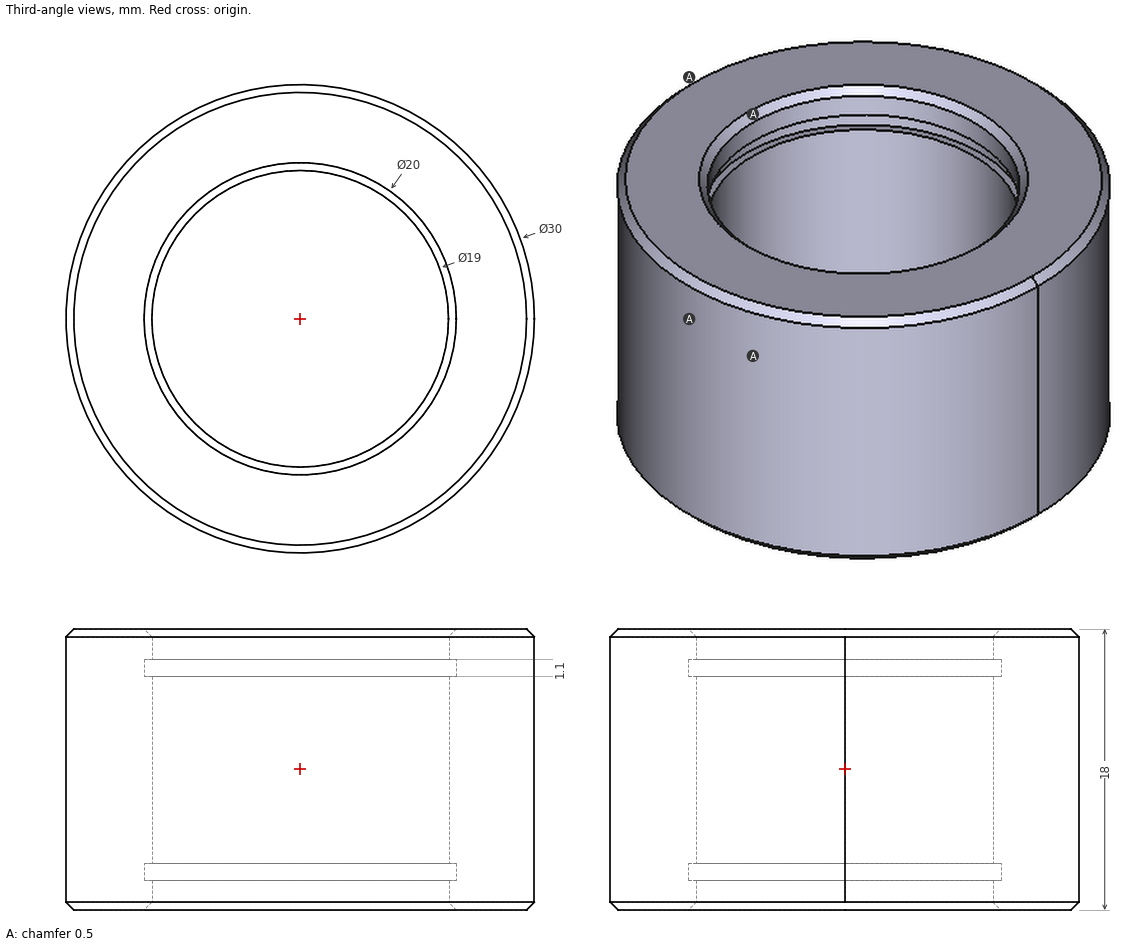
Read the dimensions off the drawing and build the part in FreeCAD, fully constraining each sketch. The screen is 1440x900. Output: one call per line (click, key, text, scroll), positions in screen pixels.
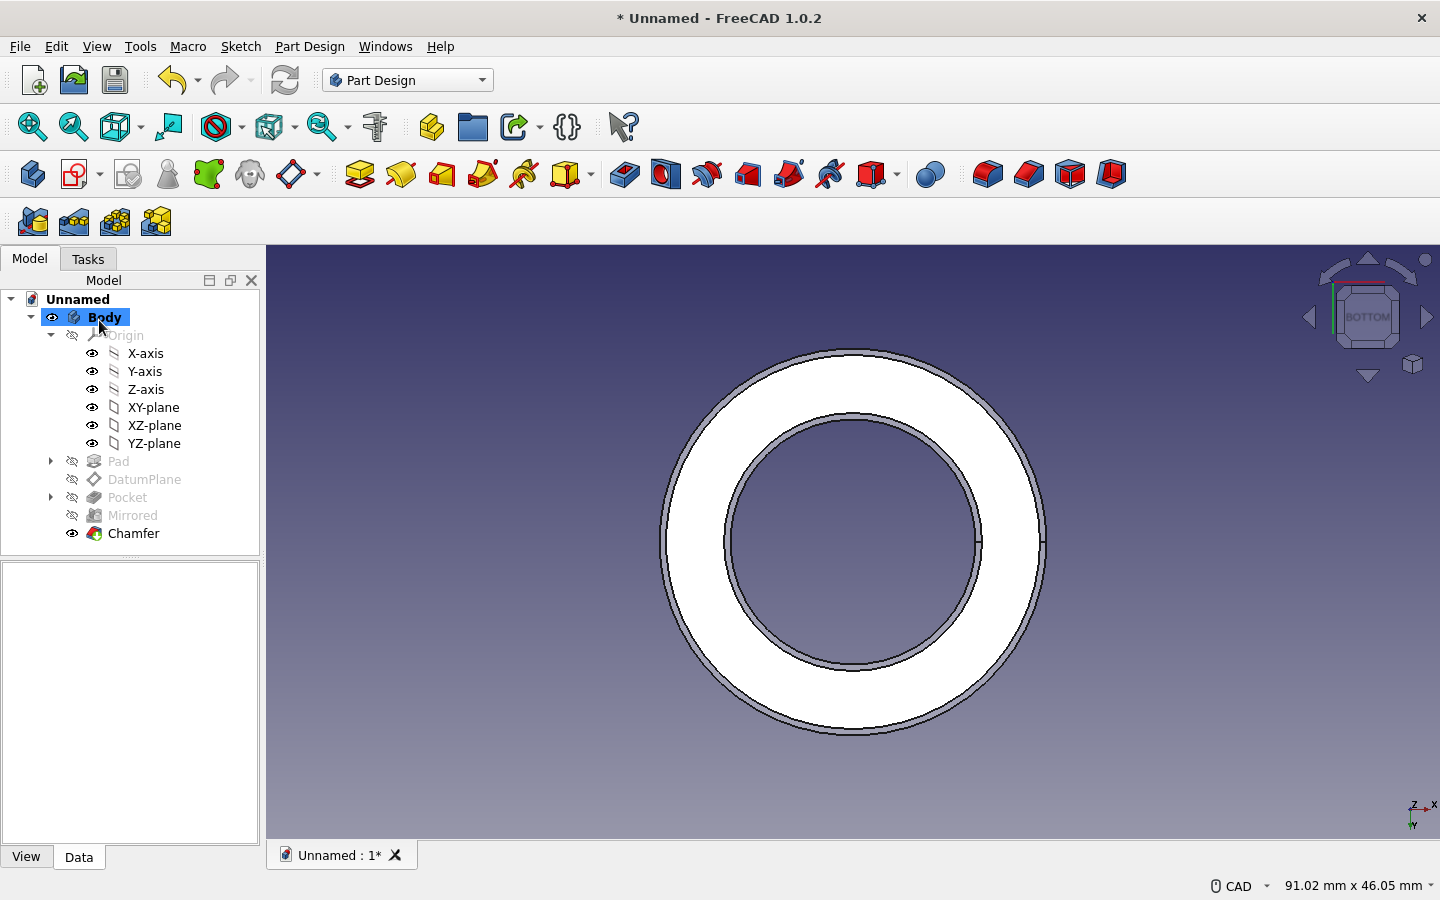
key(0)